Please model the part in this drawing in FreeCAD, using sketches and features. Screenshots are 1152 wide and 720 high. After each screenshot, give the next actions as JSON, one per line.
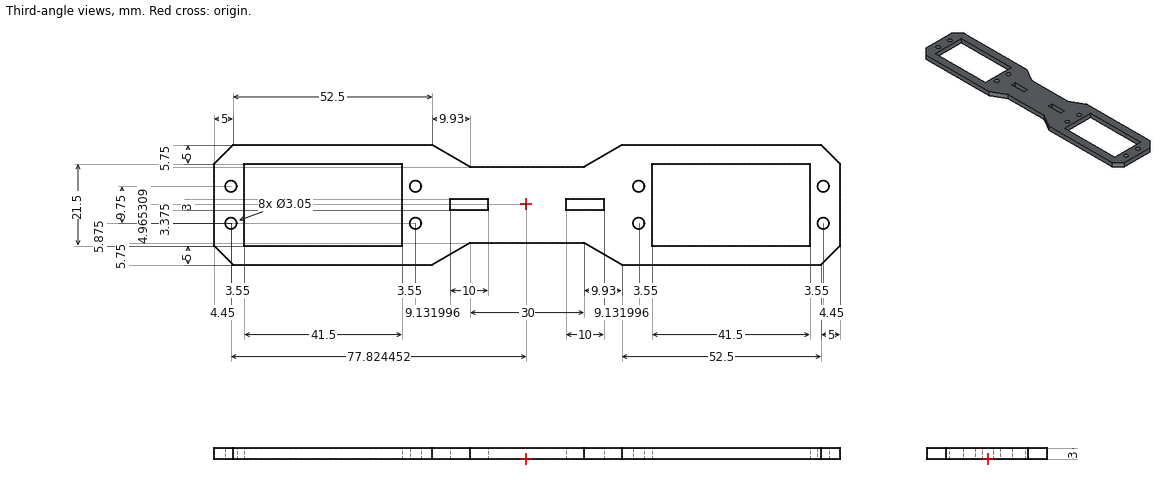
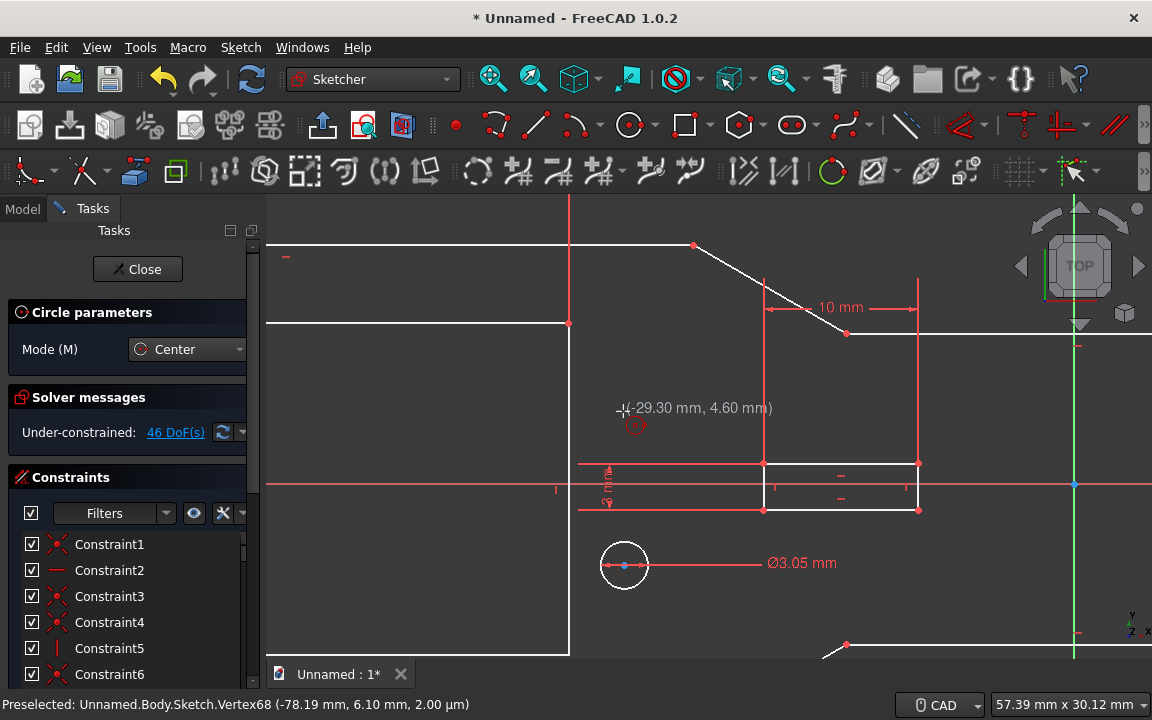
{"action": "scroll", "coordinate": [530, 412], "scroll_direction": "down", "scroll_amount": 8}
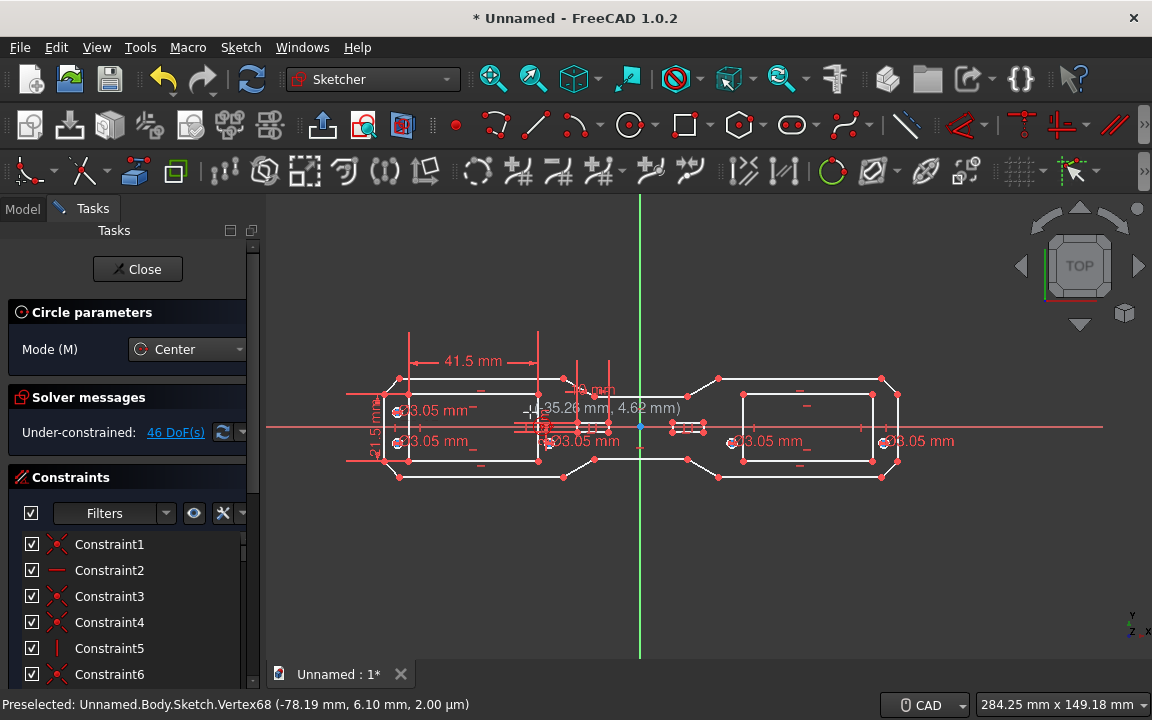
{"action": "scroll", "coordinate": [549, 412], "scroll_direction": "up", "scroll_amount": 2}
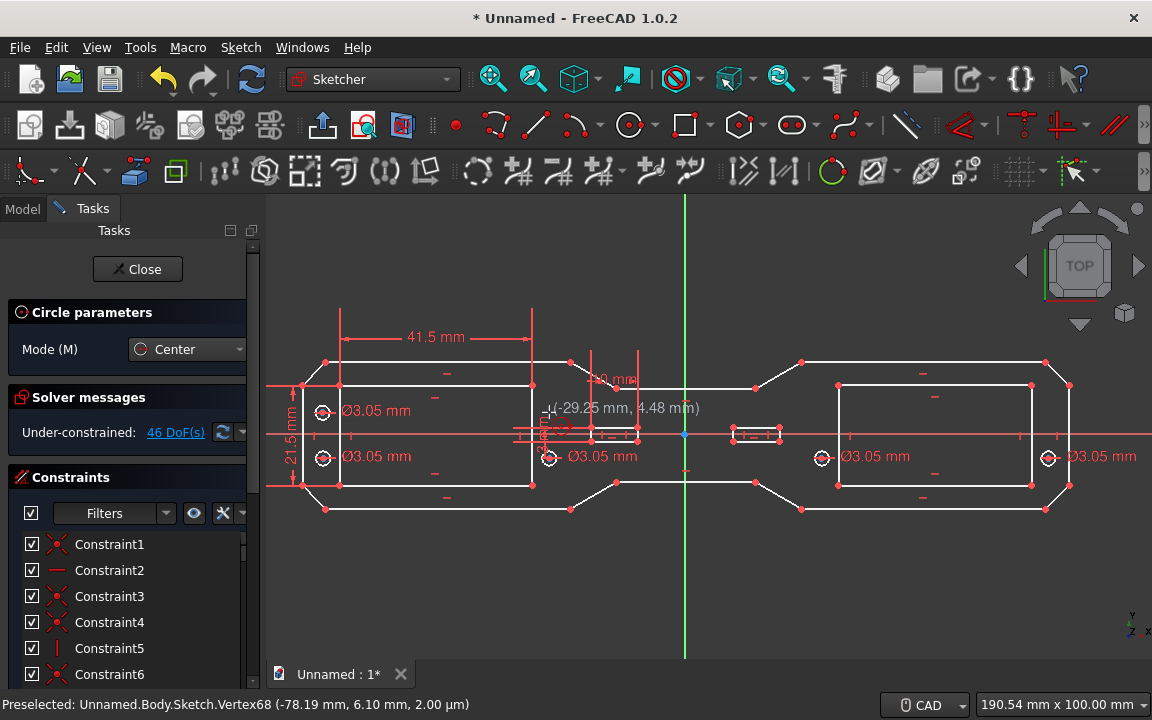
{"action": "left_click", "coordinate": [549, 412]}
{"action": "mouse_move", "coordinate": [554, 407]}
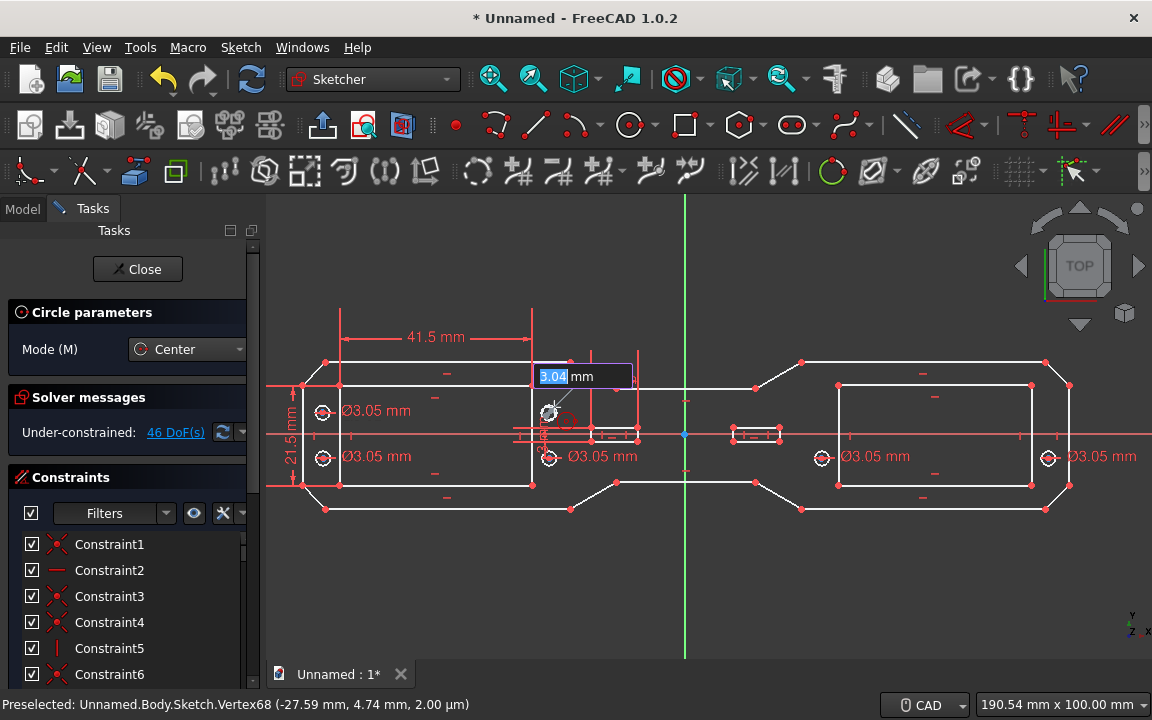
{"action": "type", "text": "3.05"}
{"action": "key", "text": "Return"}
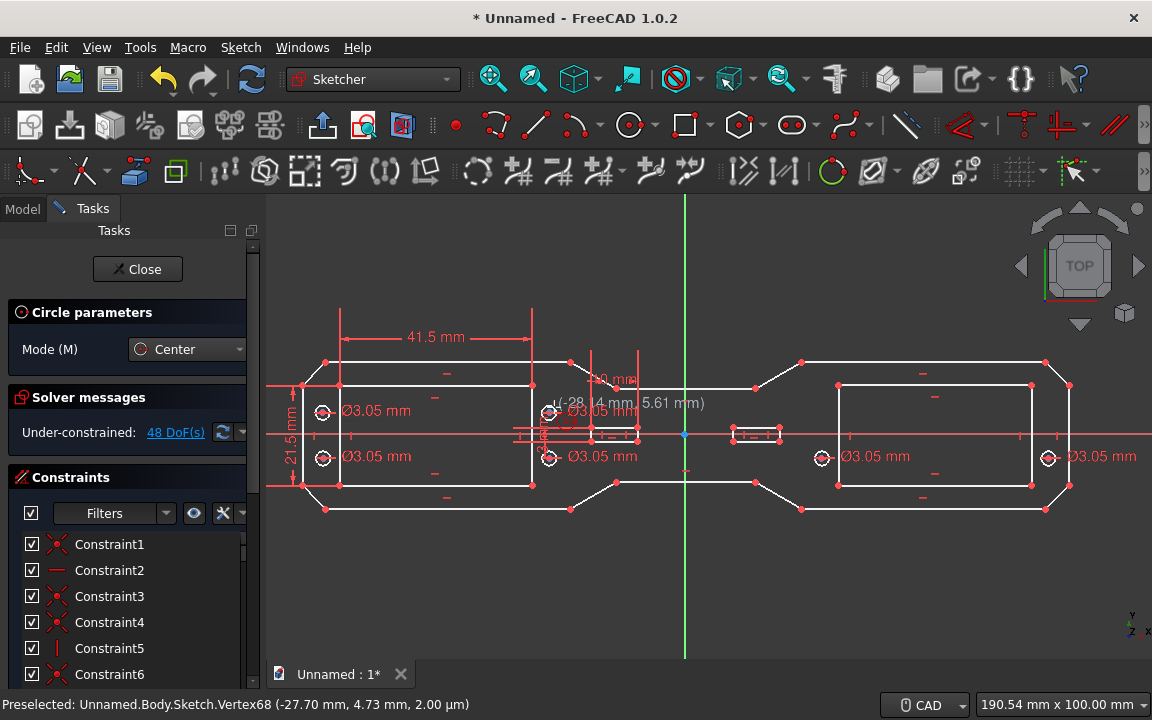
{"action": "scroll", "coordinate": [822, 412], "scroll_direction": "up", "scroll_amount": 6}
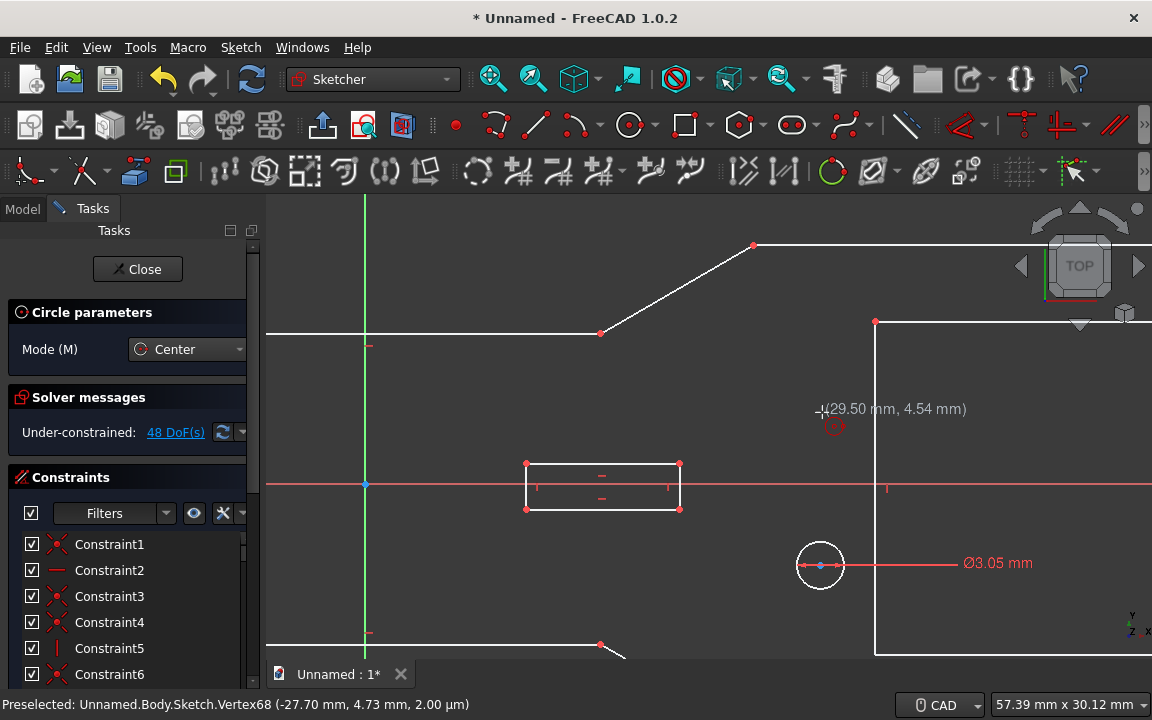
{"action": "scroll", "coordinate": [710, 412], "scroll_direction": "down", "scroll_amount": 8}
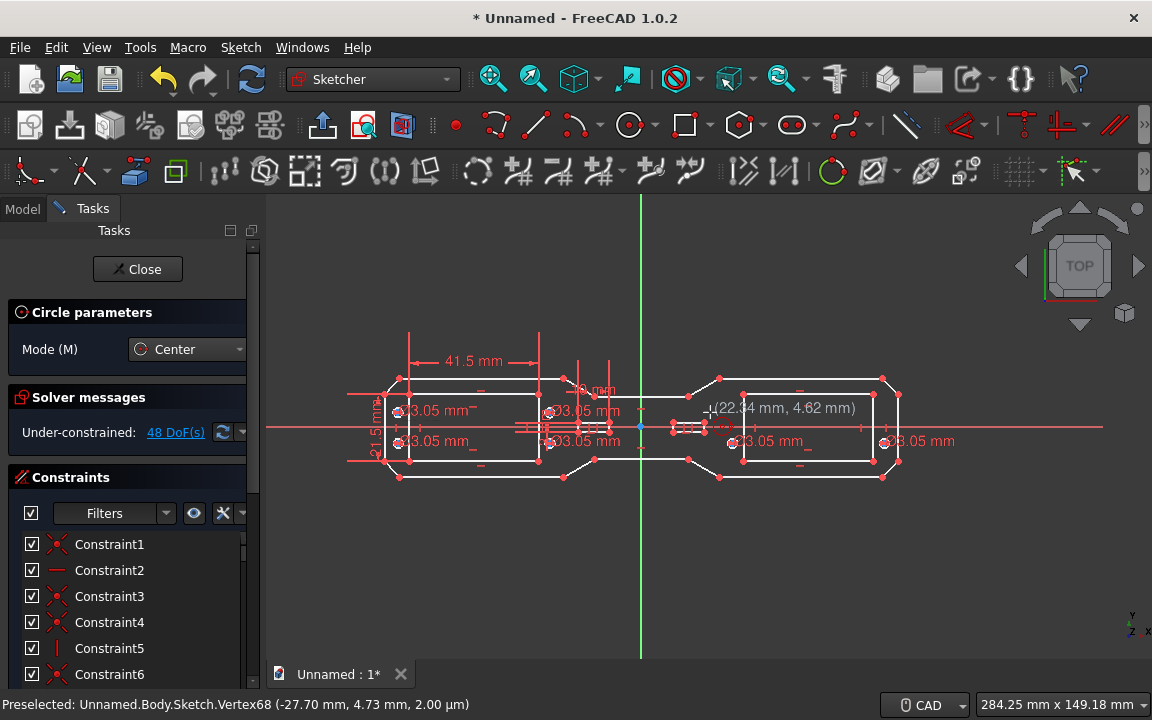
{"action": "scroll", "coordinate": [733, 412], "scroll_direction": "up", "scroll_amount": 2}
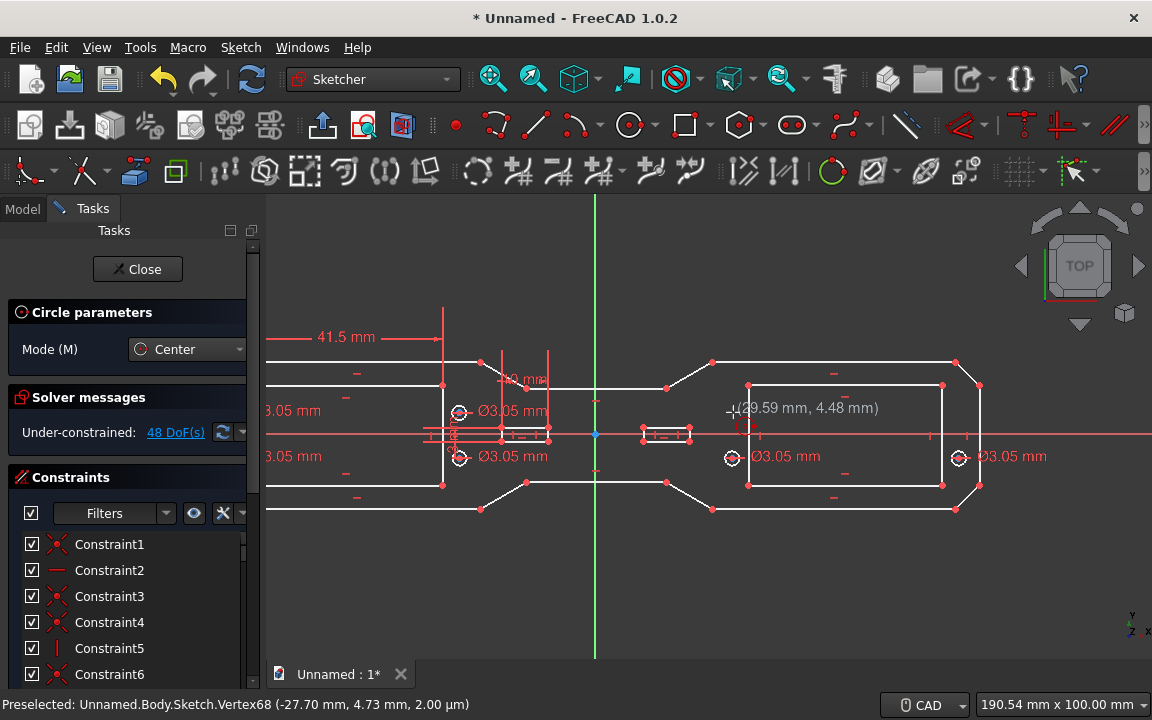
{"action": "left_click", "coordinate": [732, 412]}
{"action": "mouse_move", "coordinate": [727, 407]}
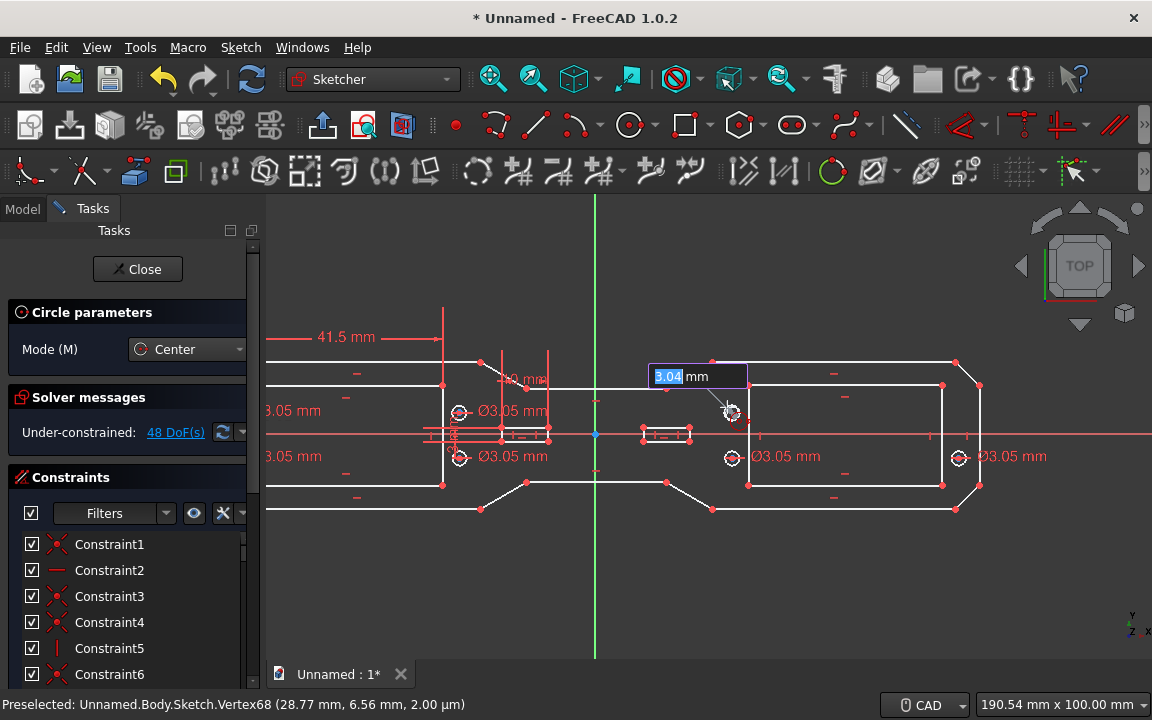
{"action": "type", "text": "3.05"}
{"action": "key", "text": "Return"}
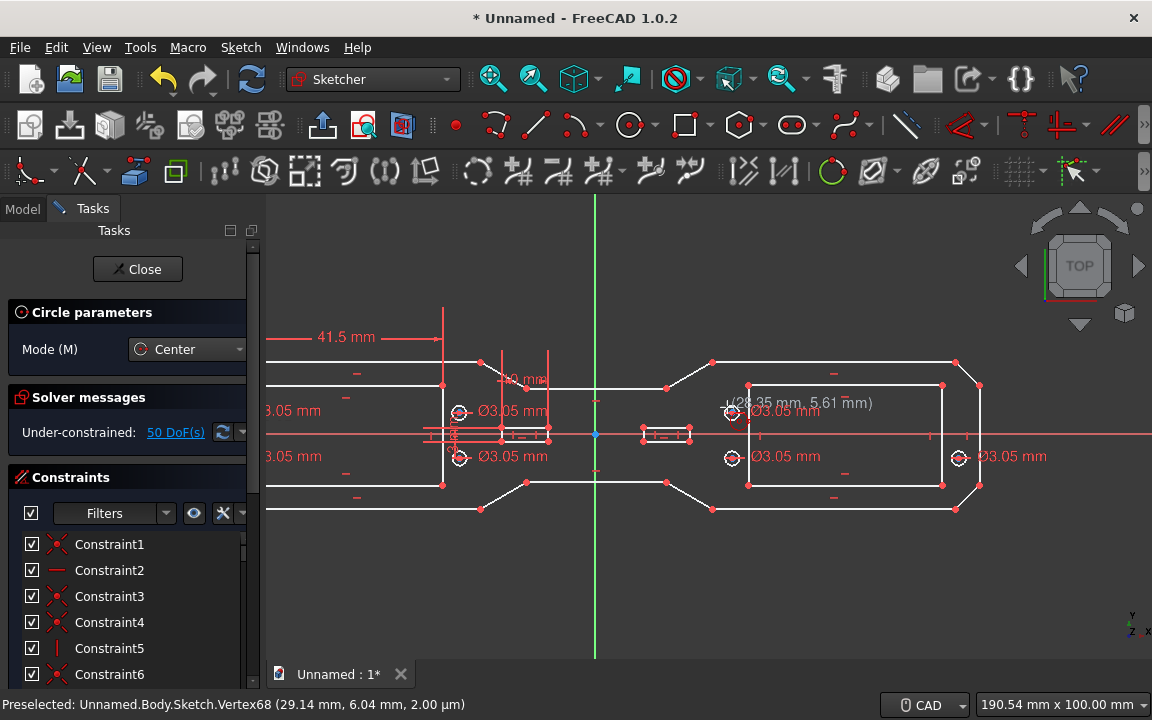
{"action": "scroll", "coordinate": [958, 412], "scroll_direction": "up", "scroll_amount": 6}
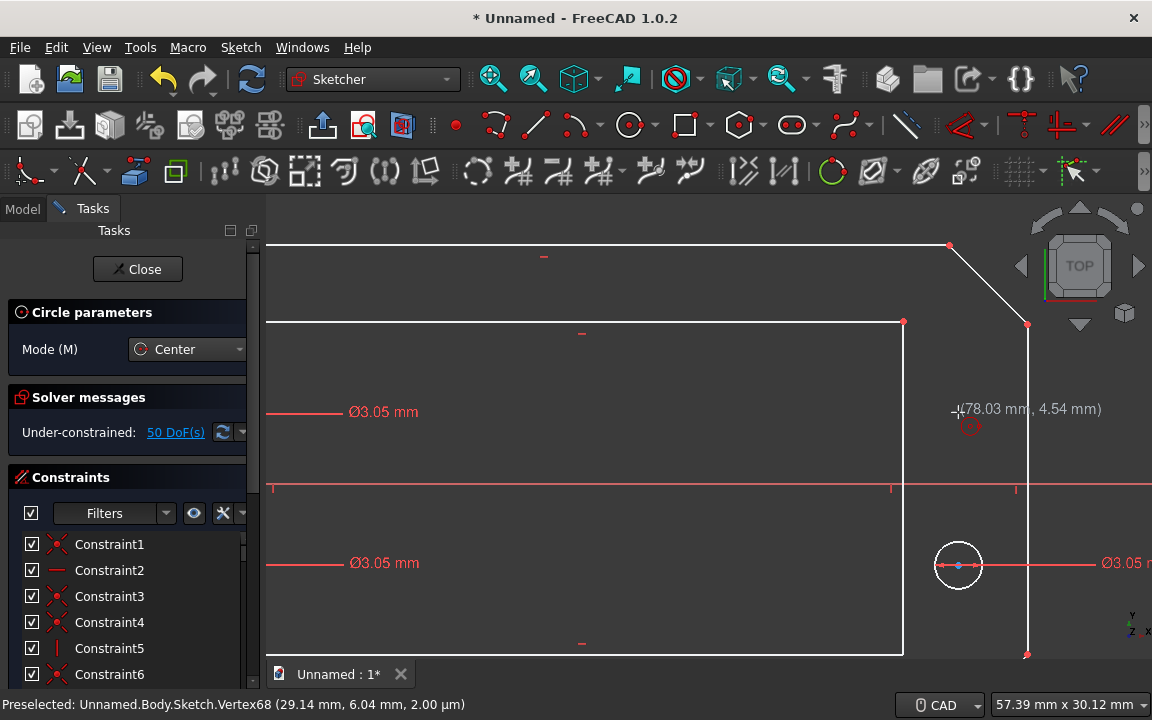
{"action": "scroll", "coordinate": [865, 412], "scroll_direction": "down", "scroll_amount": 8}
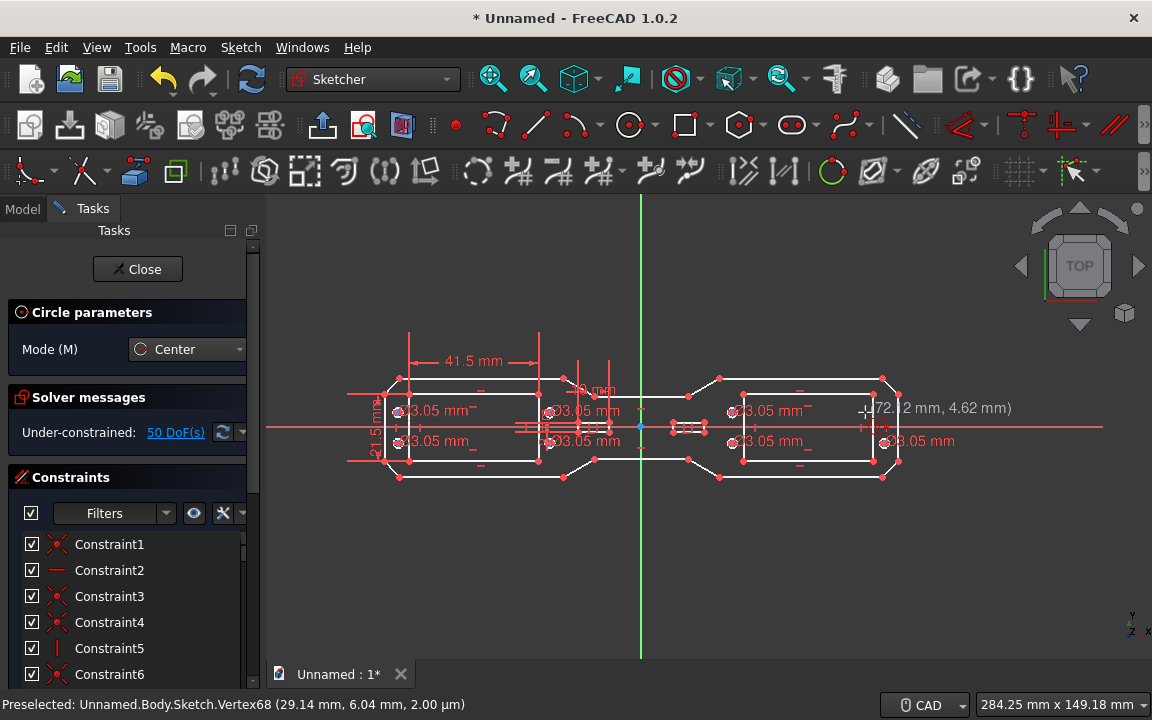
{"action": "scroll", "coordinate": [884, 412], "scroll_direction": "up", "scroll_amount": 2}